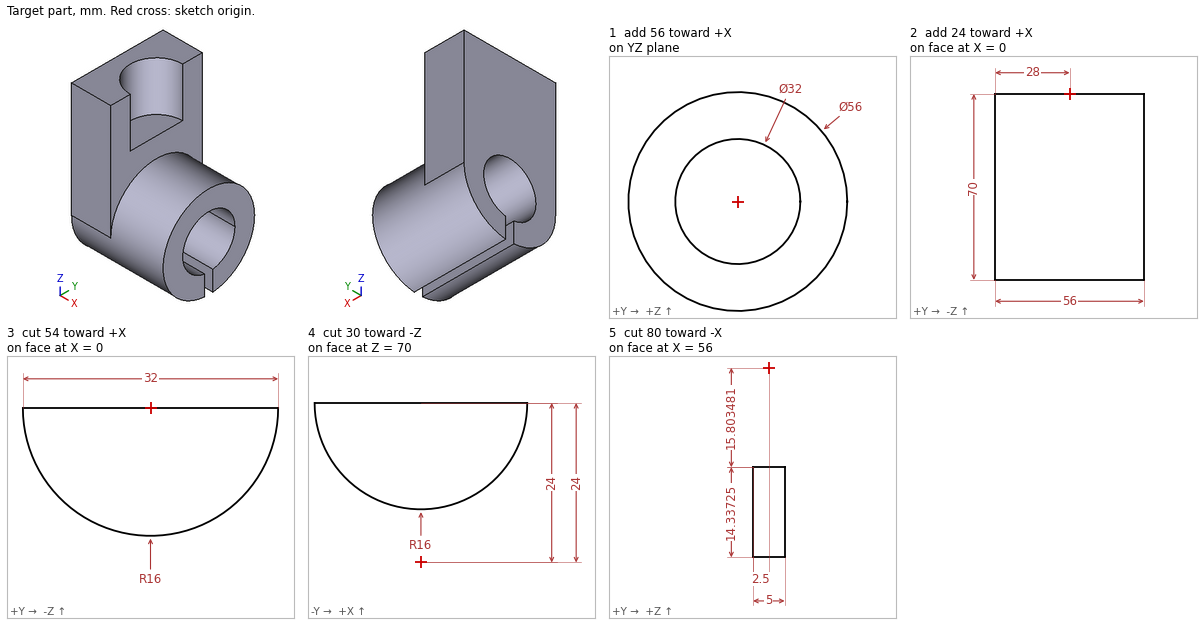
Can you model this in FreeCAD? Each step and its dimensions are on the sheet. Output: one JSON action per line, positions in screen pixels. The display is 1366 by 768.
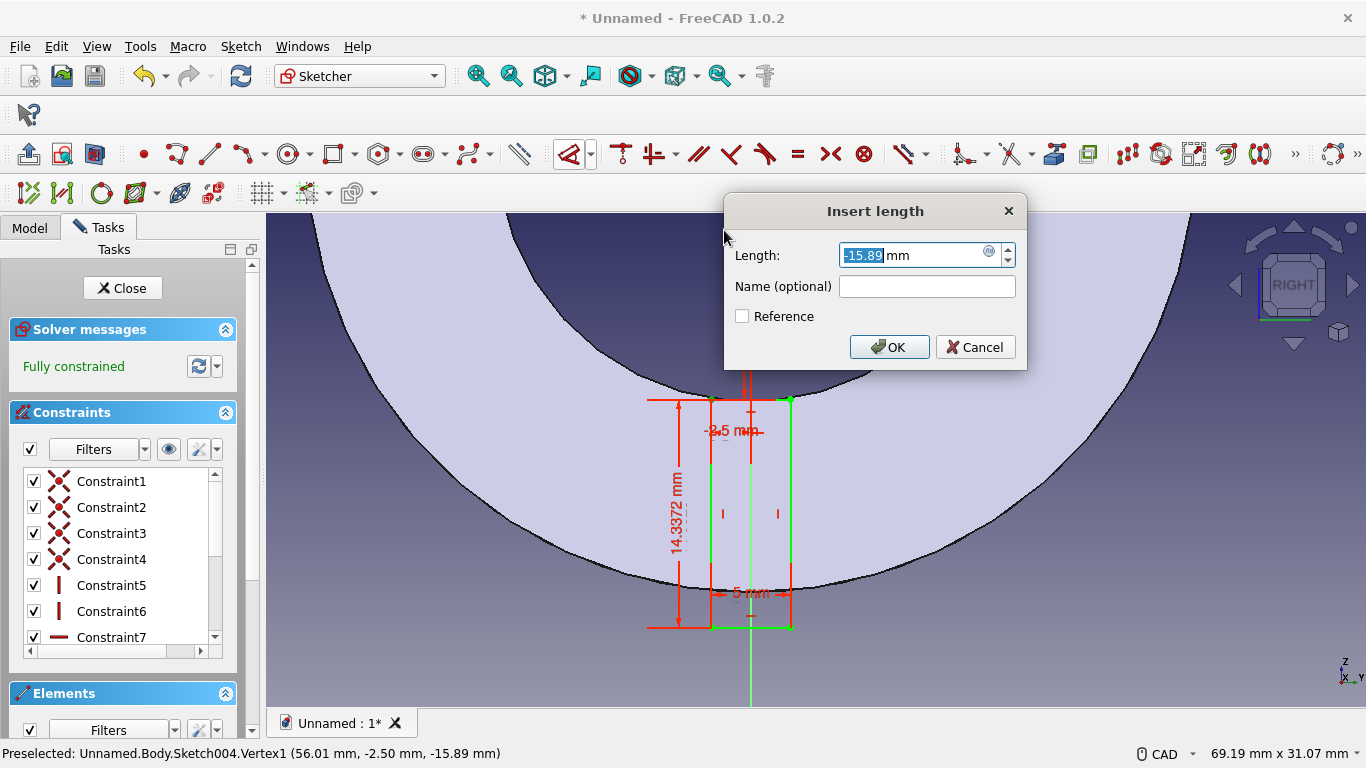
{"action": "type", "text": "-15.803481"}
{"action": "key", "text": "Return"}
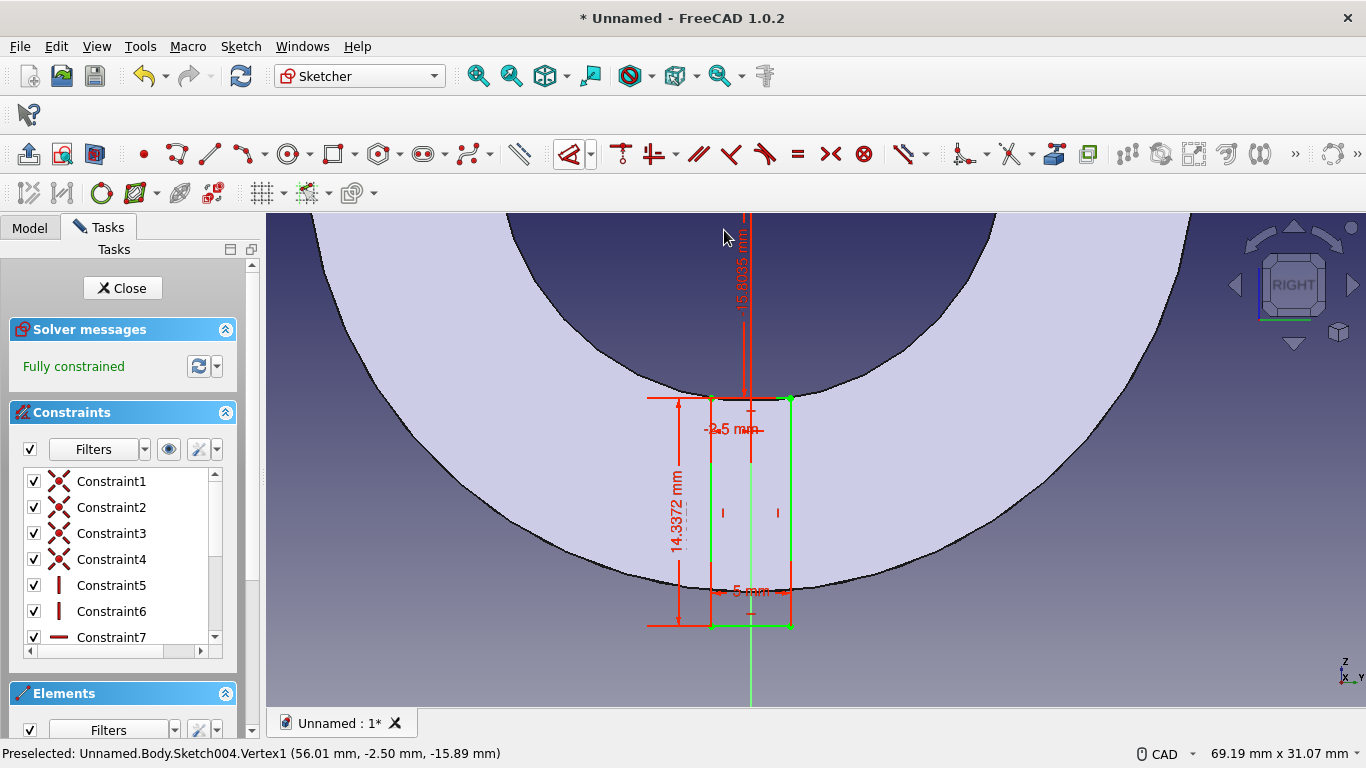
{"action": "left_click", "coordinate": [123, 288]}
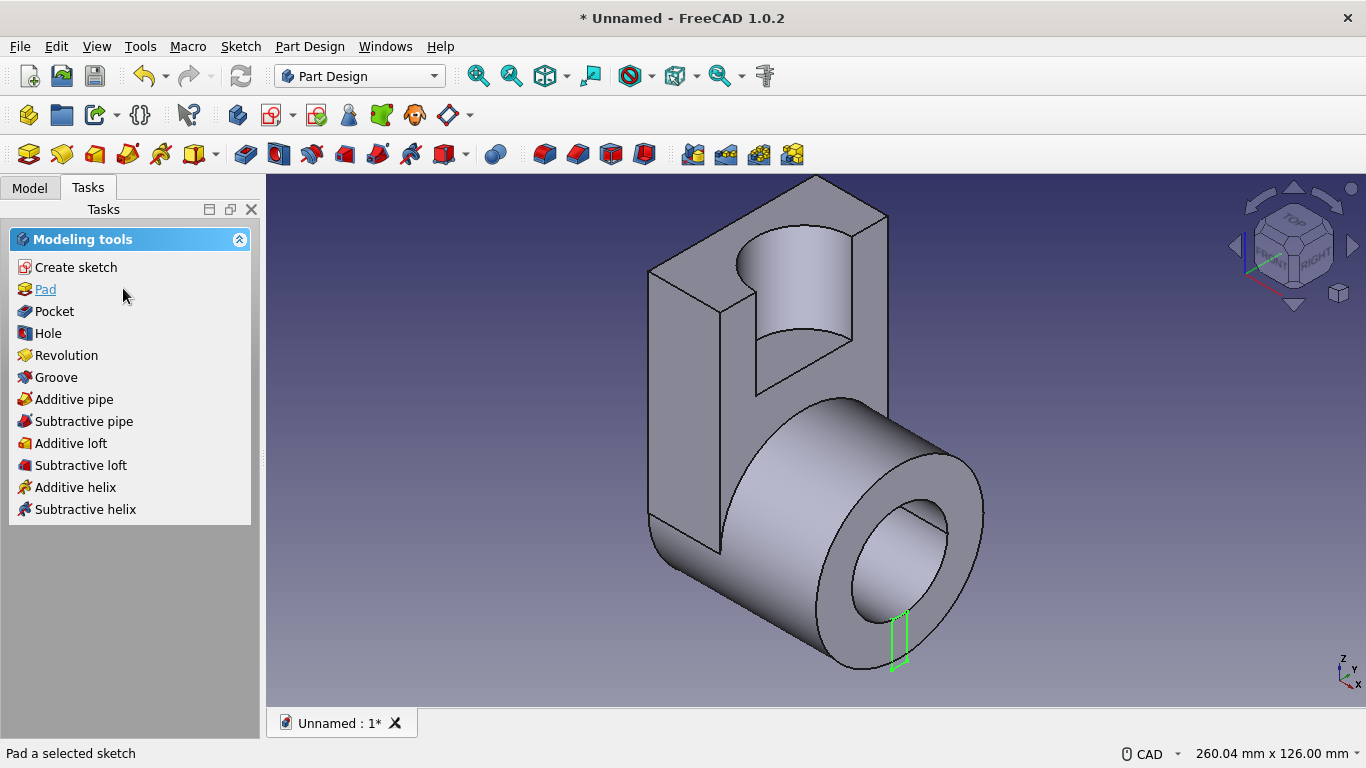
{"action": "left_click", "coordinate": [246, 154]}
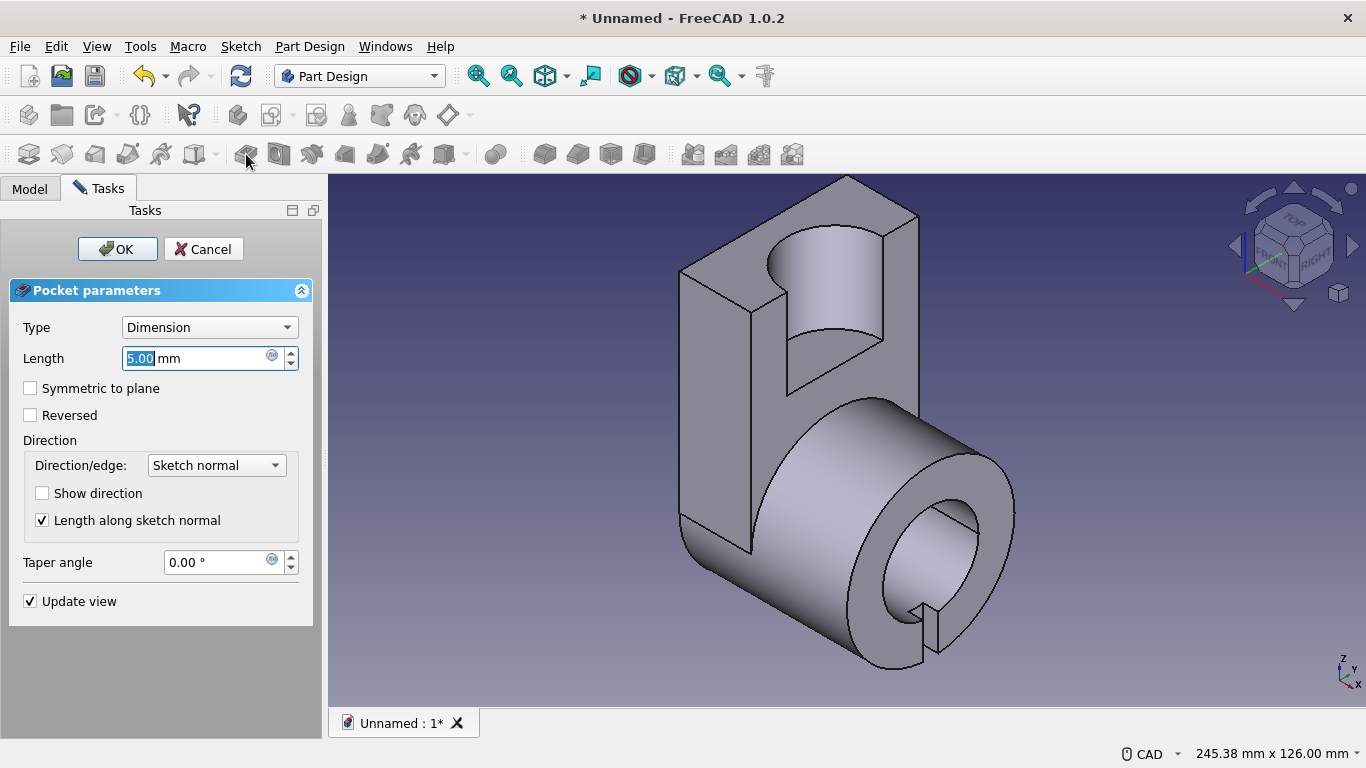
{"action": "type", "text": "80"}
{"action": "key", "text": "Tab"}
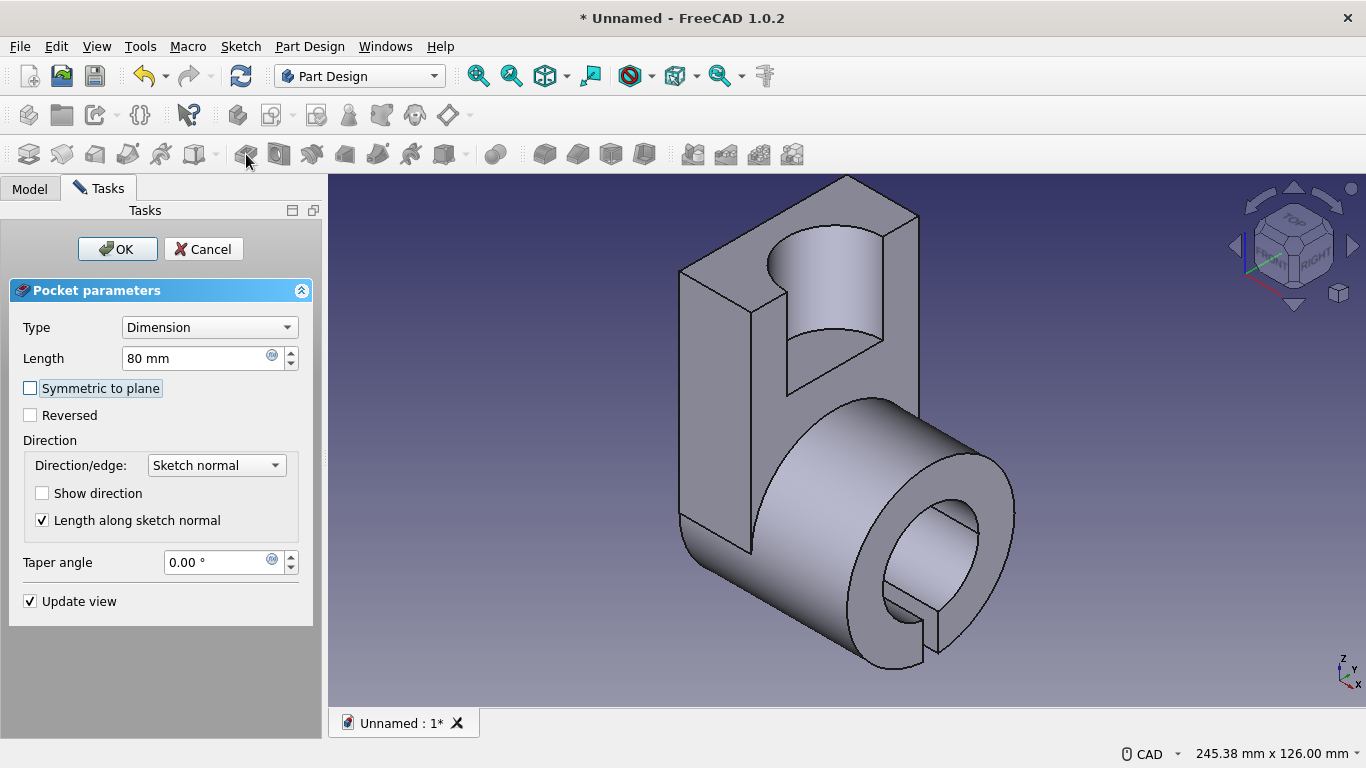
{"action": "left_click", "coordinate": [118, 249]}